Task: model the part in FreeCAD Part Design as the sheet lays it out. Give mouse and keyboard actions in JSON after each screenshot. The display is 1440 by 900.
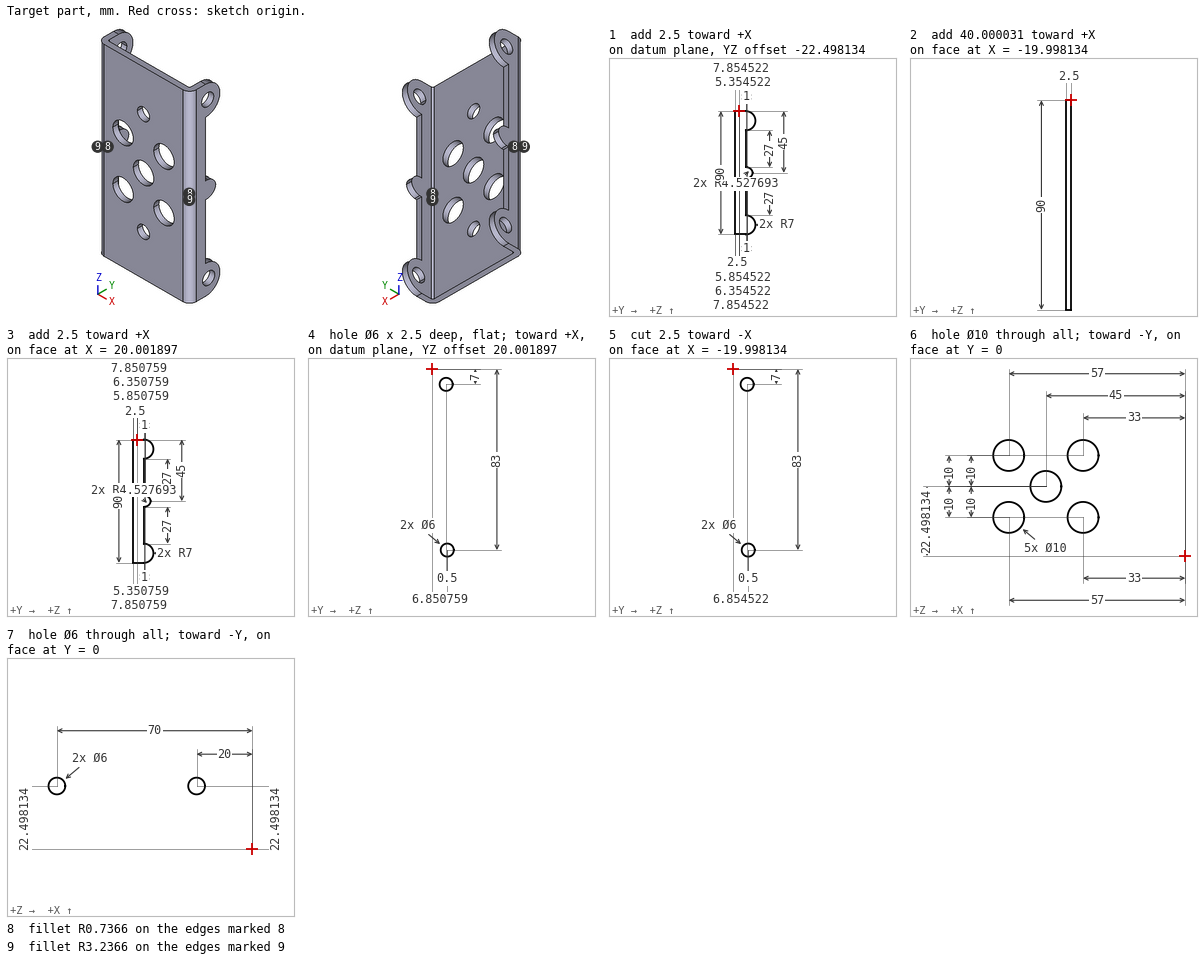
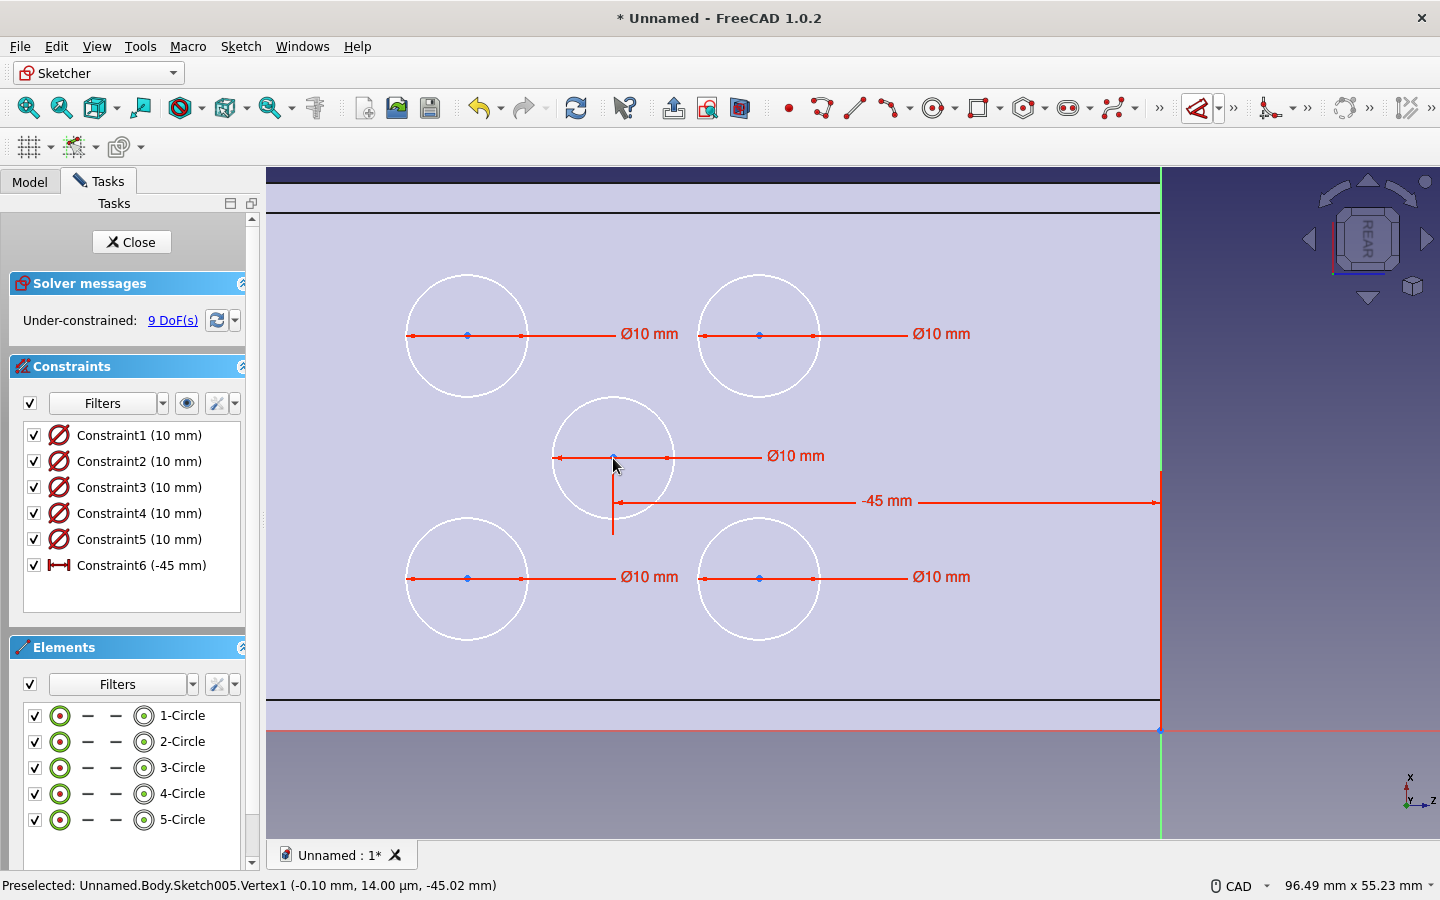
{"action": "left_click", "coordinate": [467, 579]}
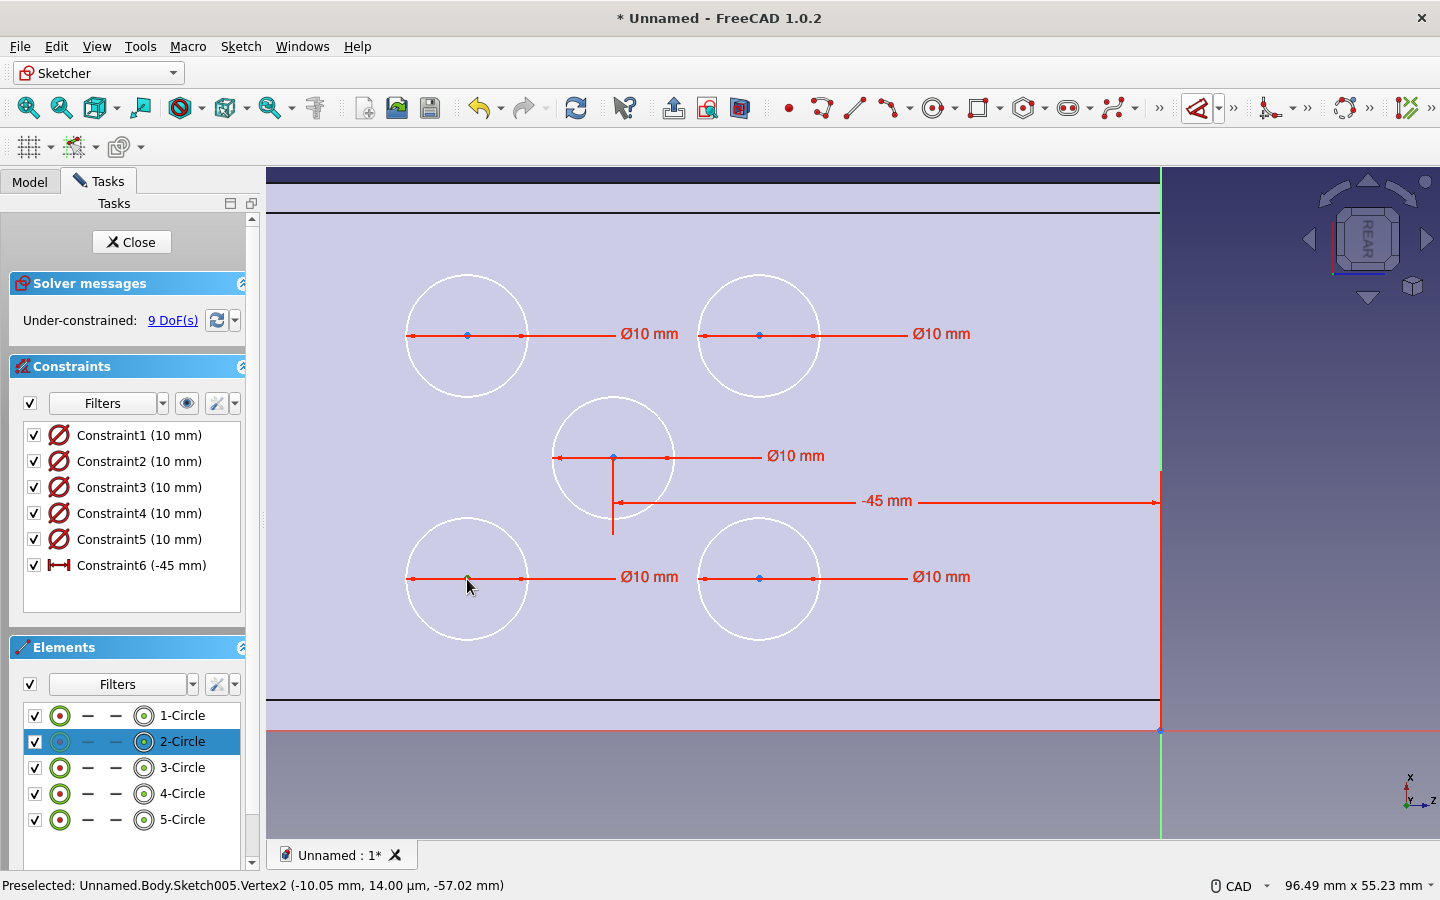
{"action": "left_click", "coordinate": [1218, 108]}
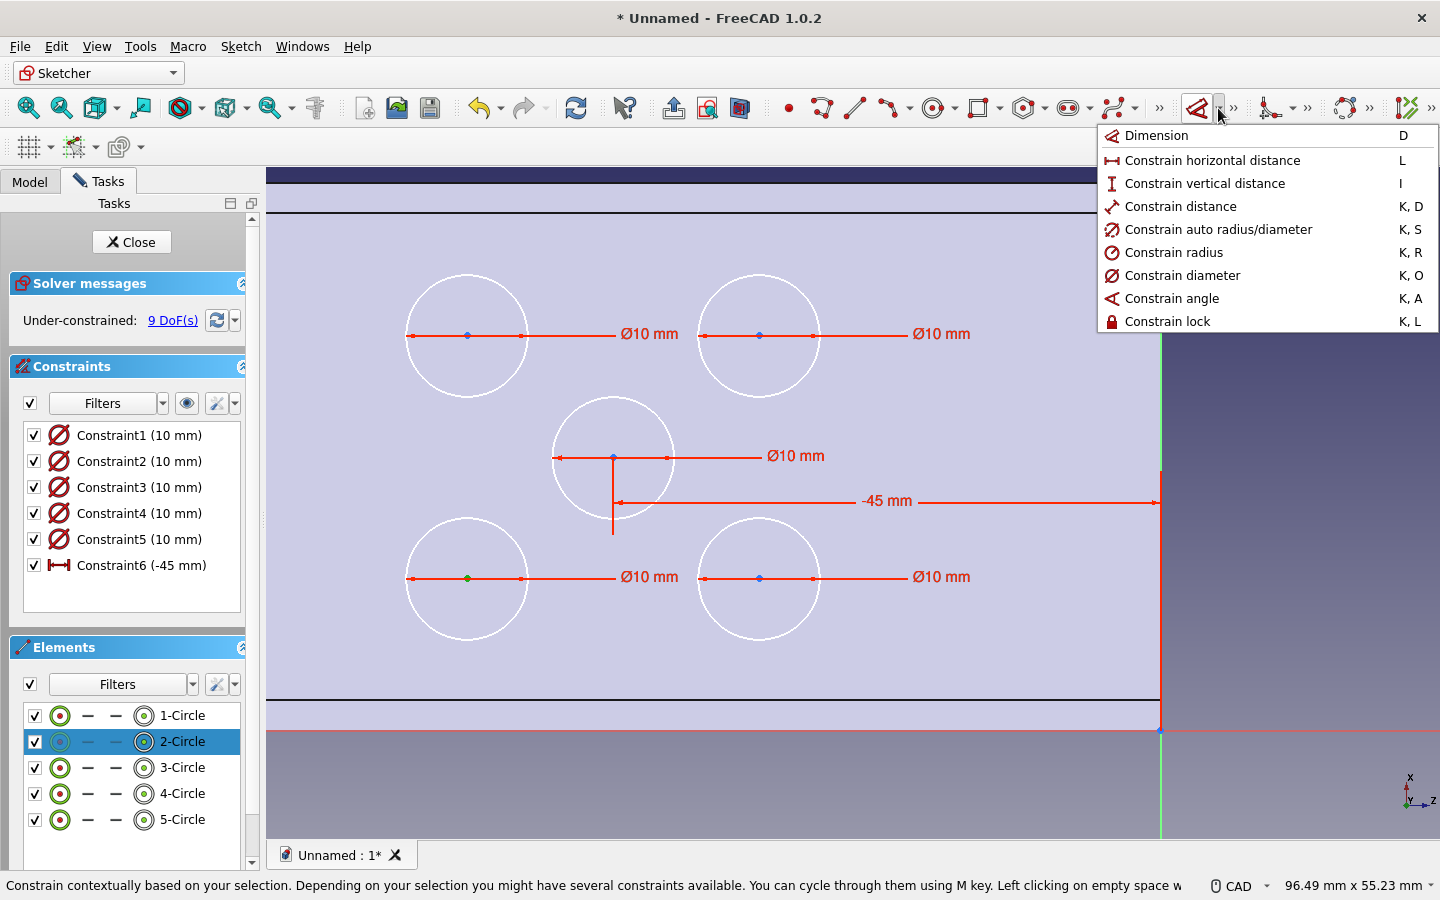
{"action": "left_click", "coordinate": [1268, 160]}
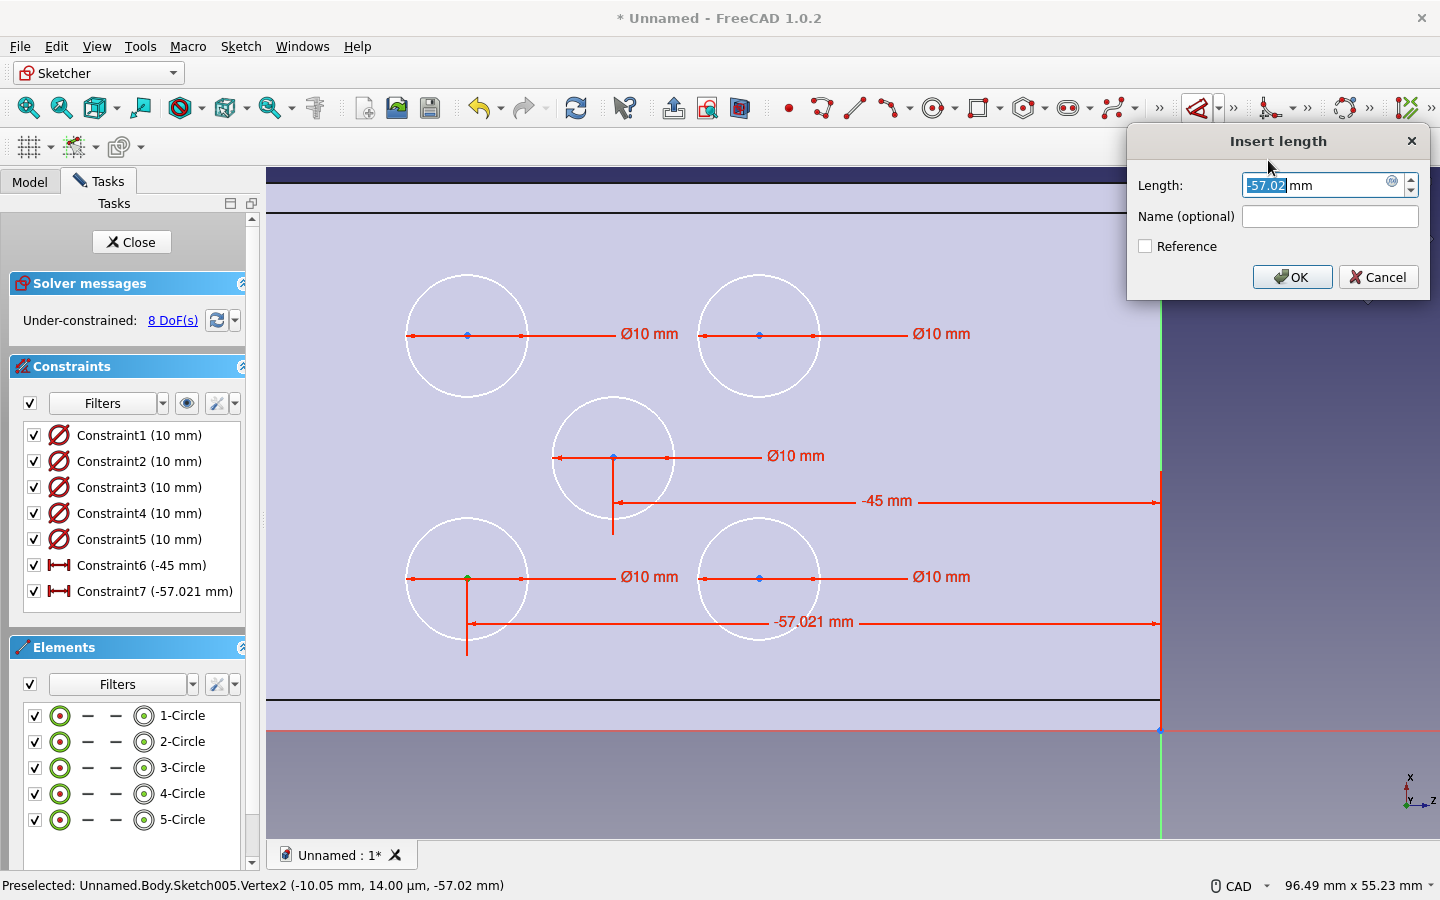
{"action": "type", "text": "-57"}
{"action": "key", "text": "Return"}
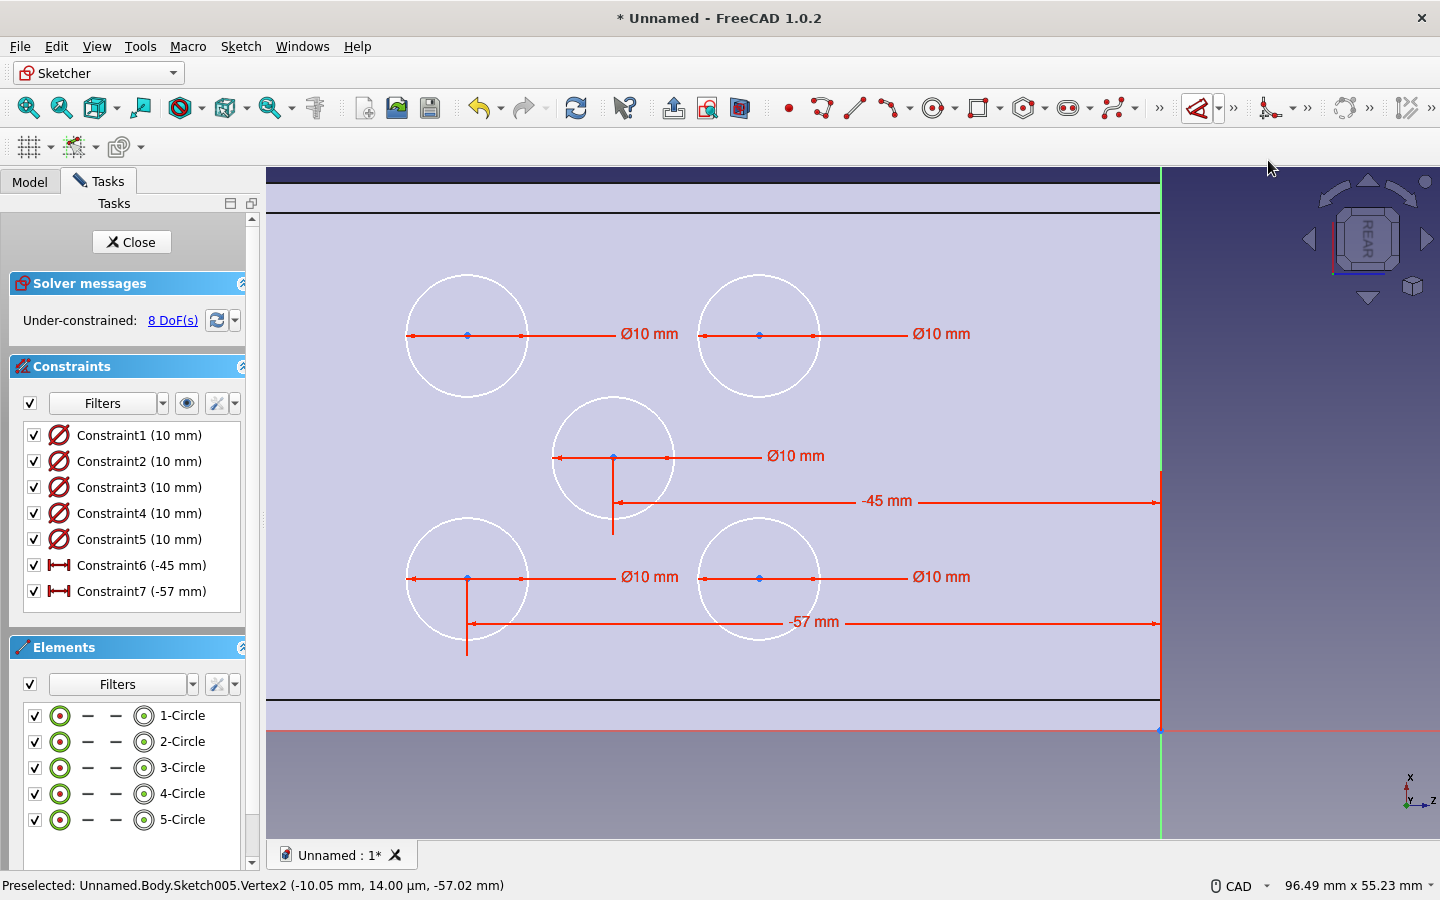
{"action": "left_click", "coordinate": [759, 579]}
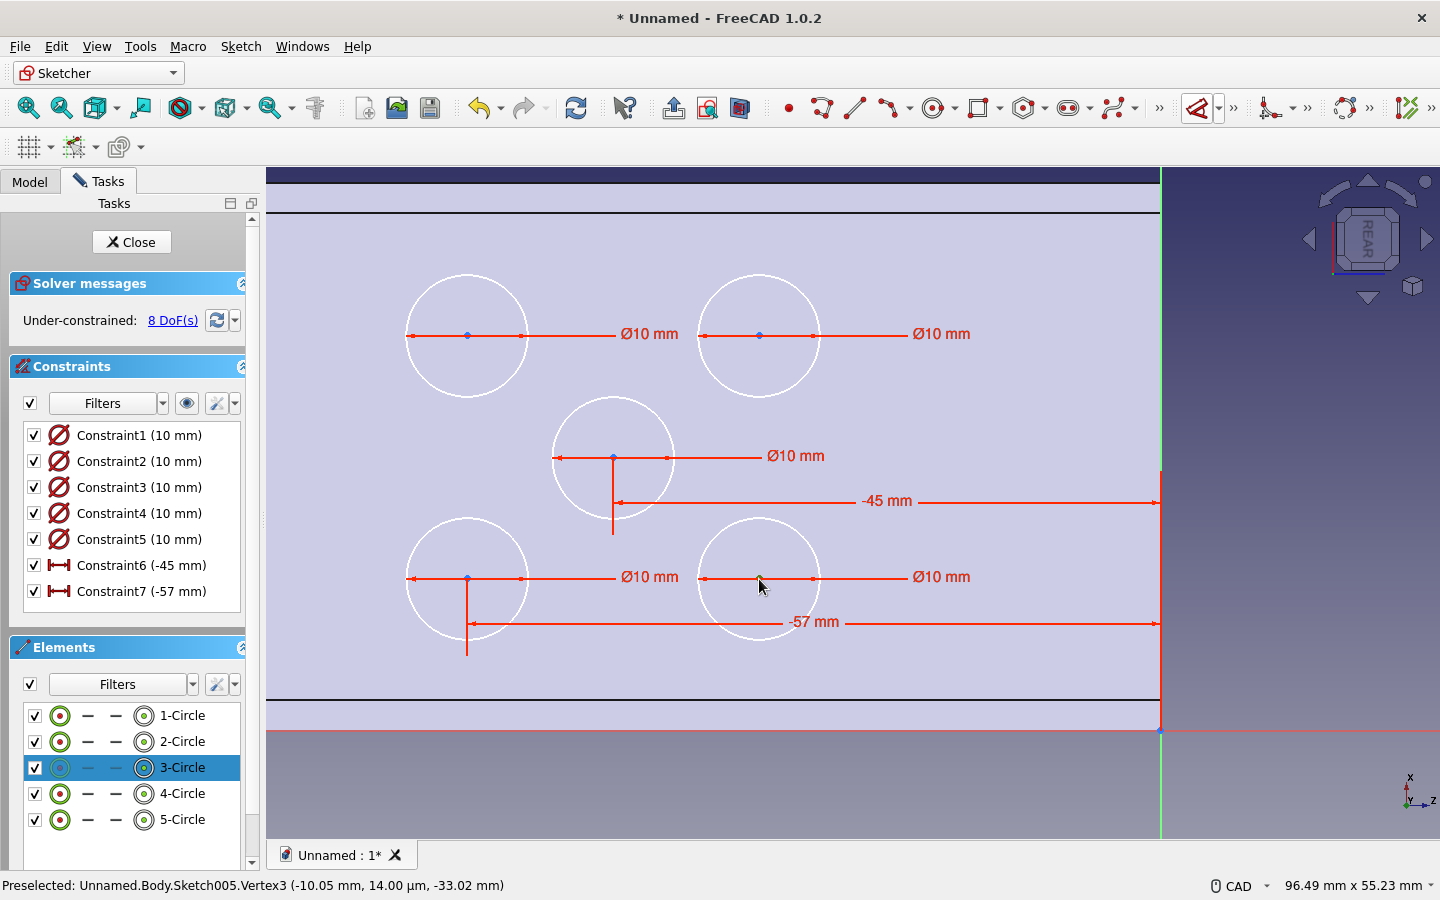
{"action": "left_click", "coordinate": [1218, 108]}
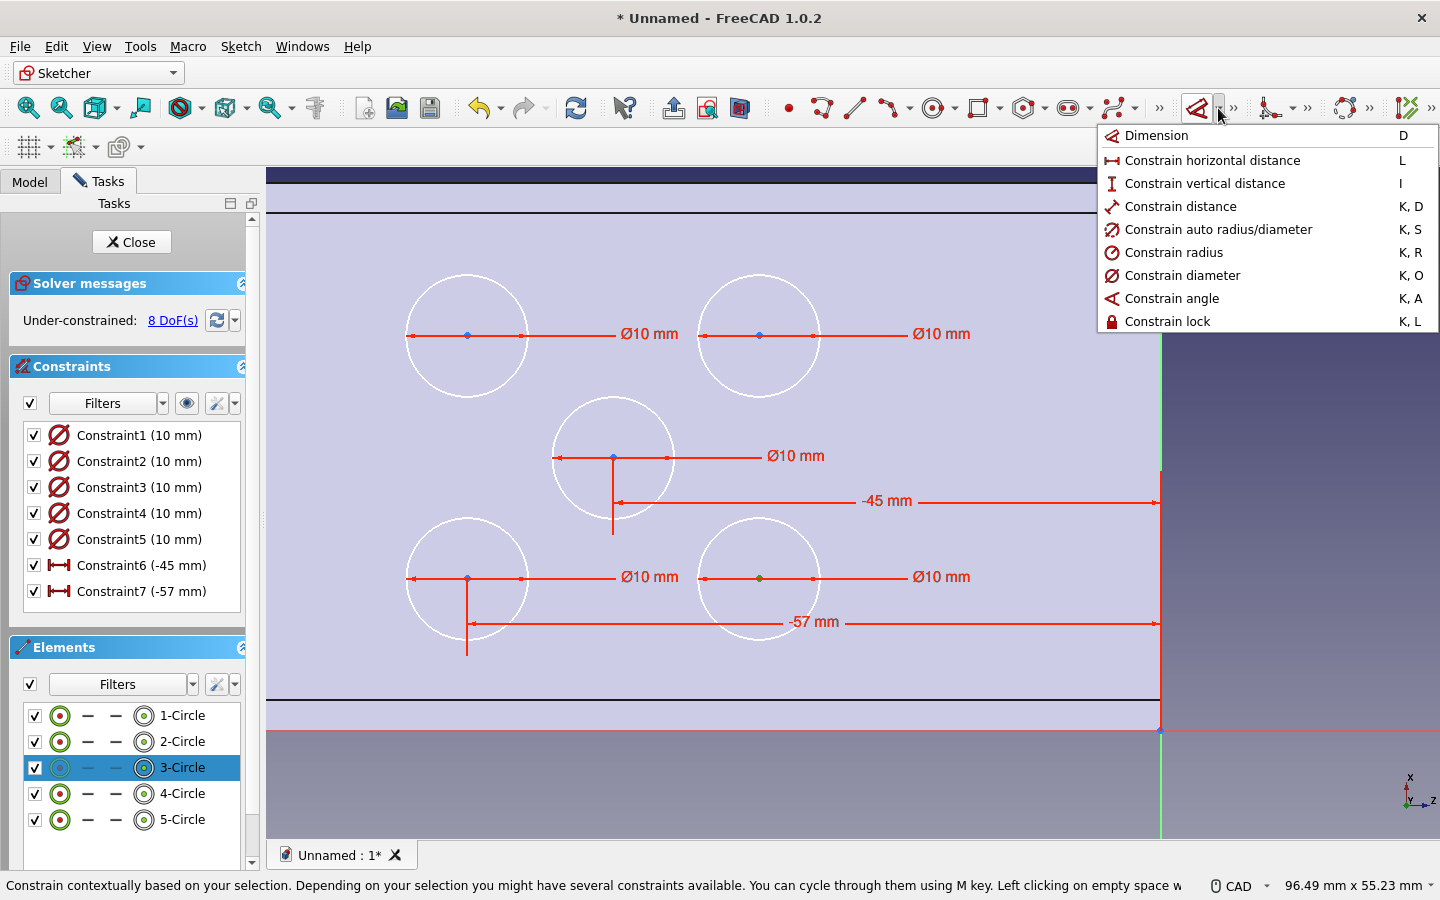
{"action": "left_click", "coordinate": [1268, 160]}